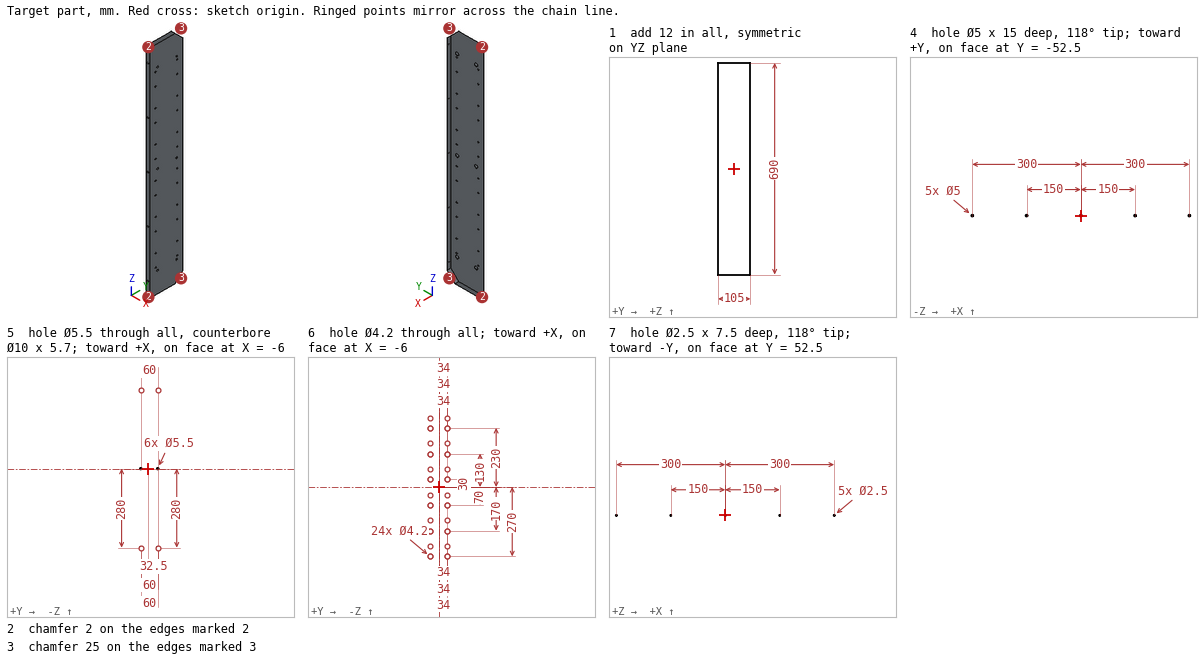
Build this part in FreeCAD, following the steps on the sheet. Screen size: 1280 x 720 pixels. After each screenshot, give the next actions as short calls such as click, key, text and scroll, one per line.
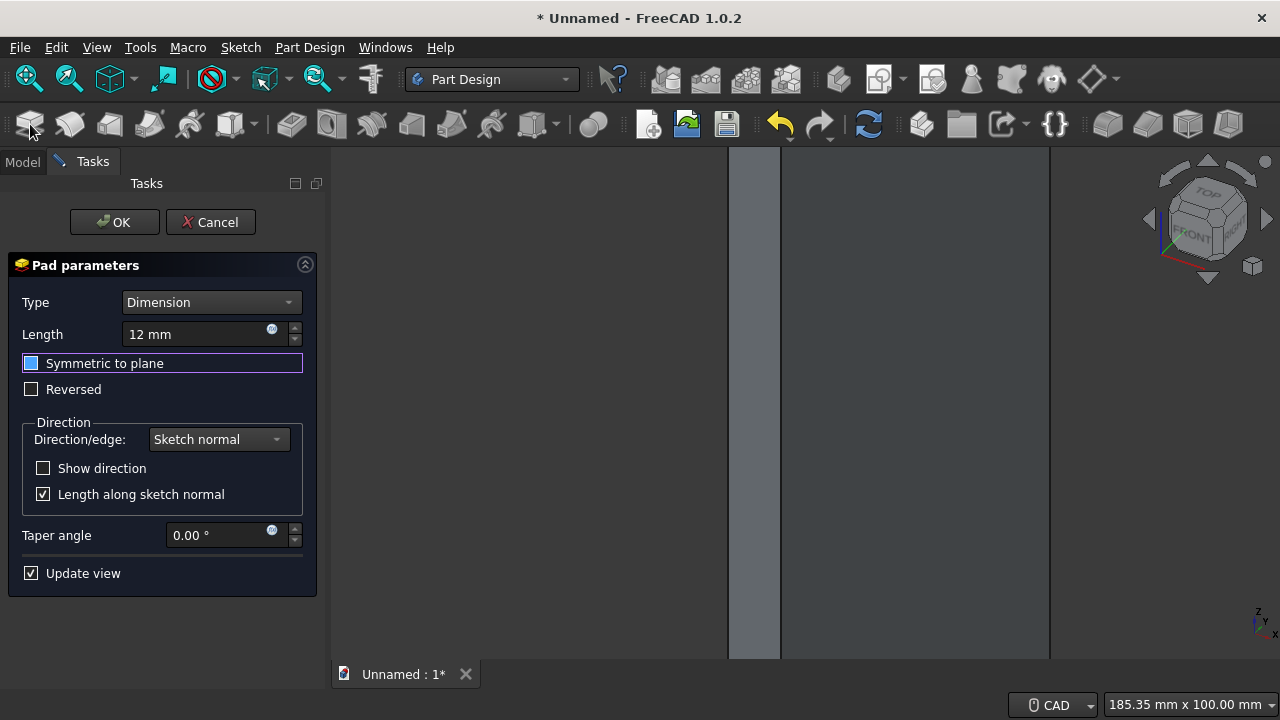
click(30, 363)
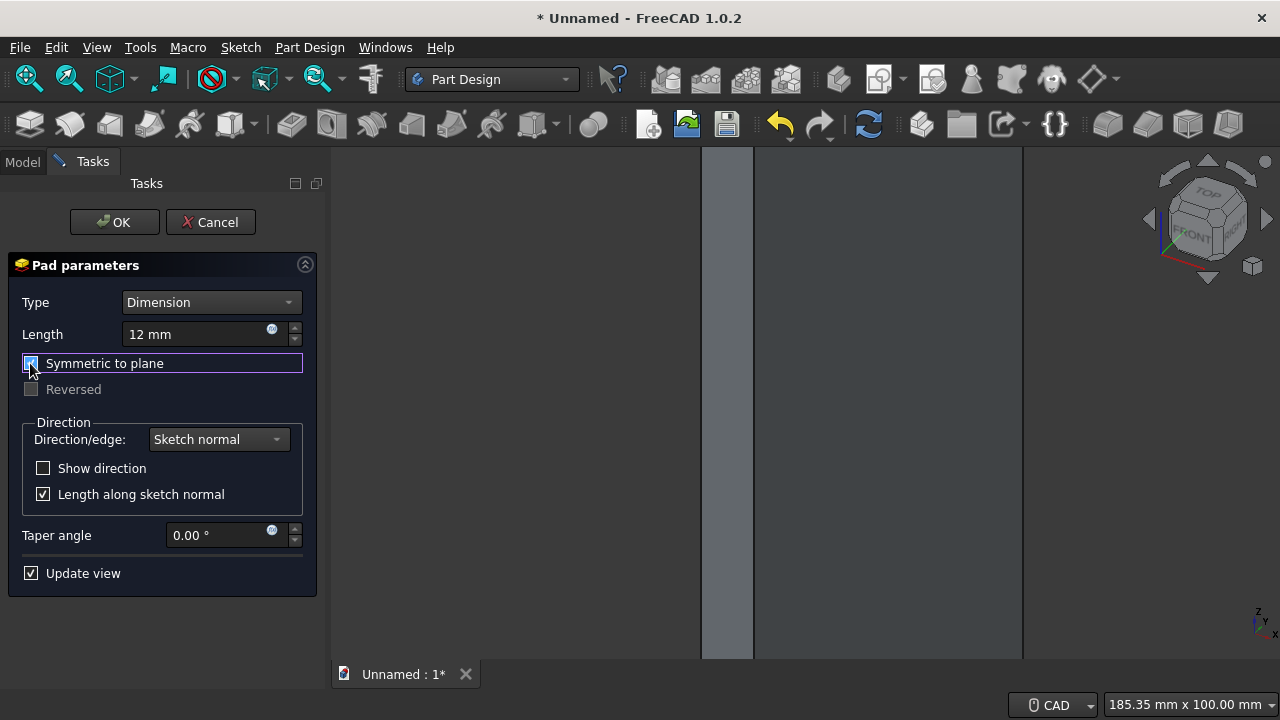
click(115, 222)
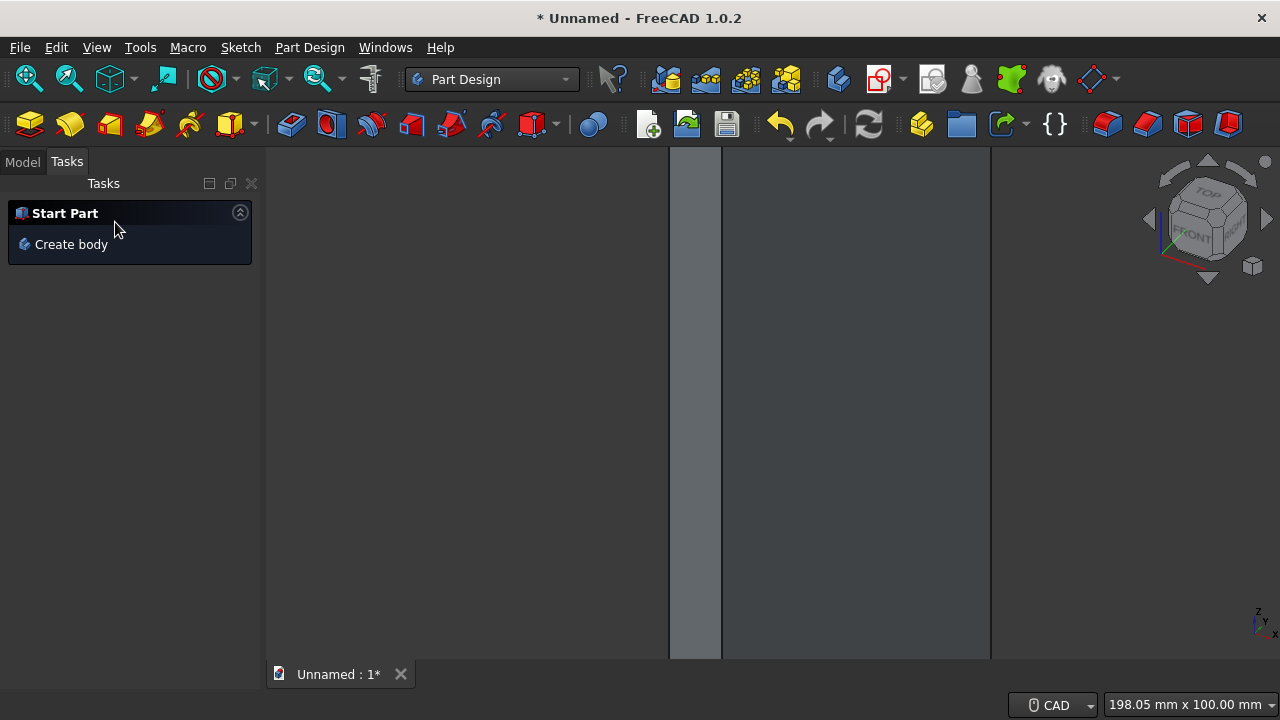
key(v)
key(f)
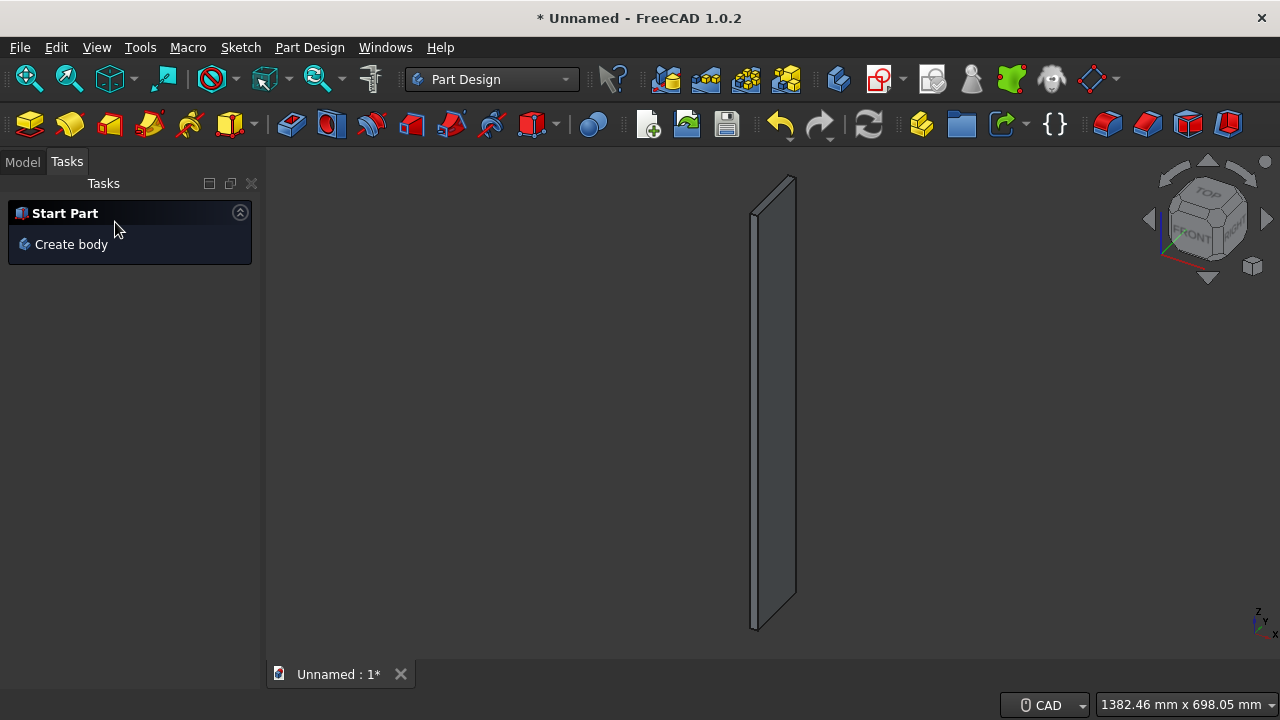
scroll(754, 628, up, 8)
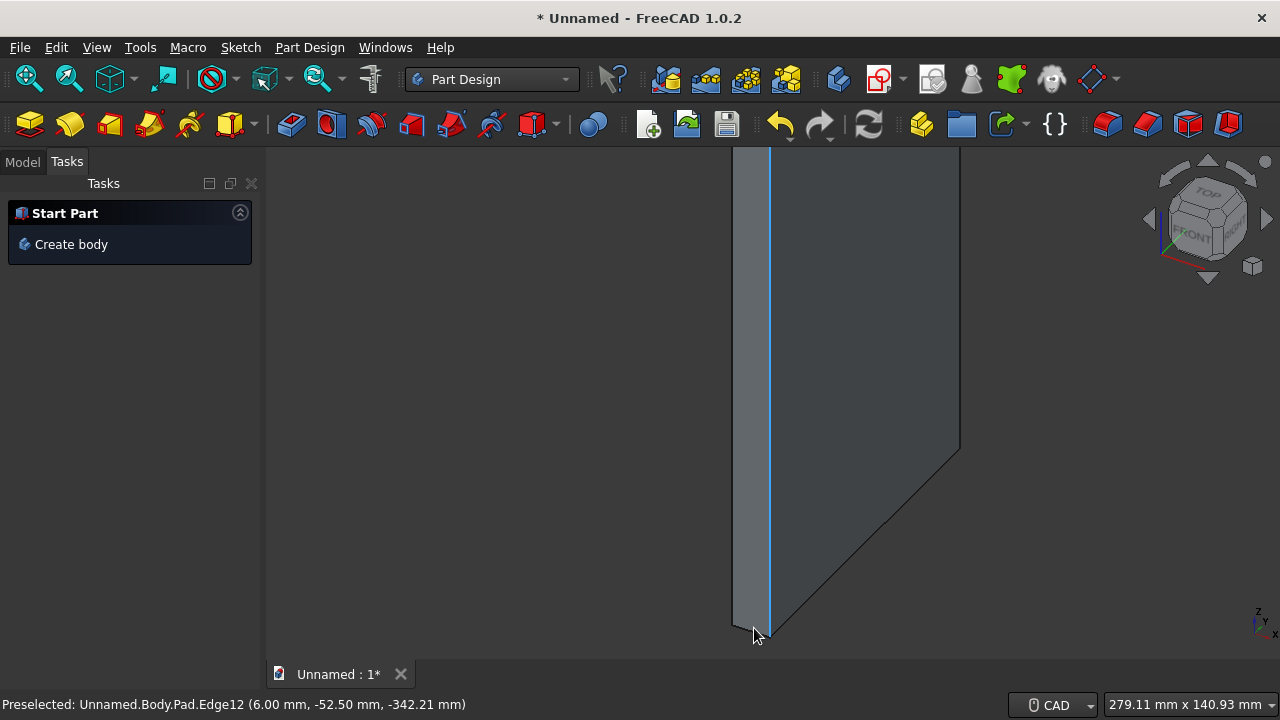
click(30, 80)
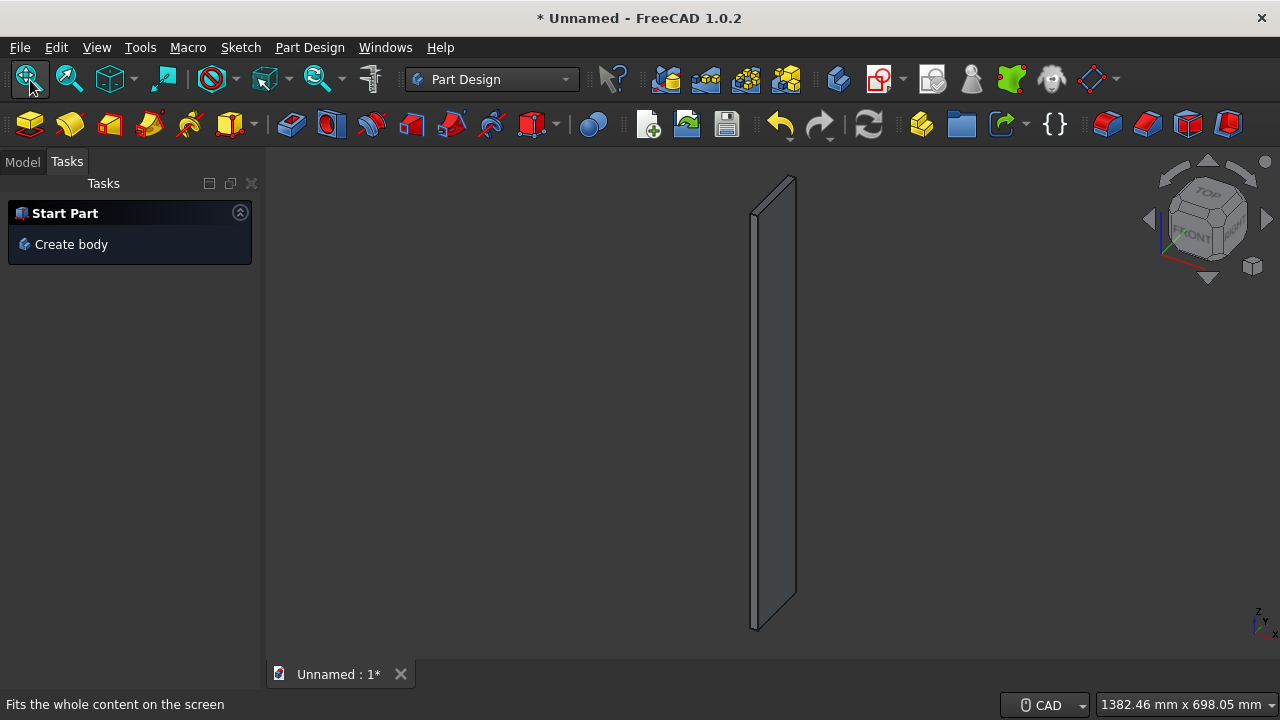
key(0)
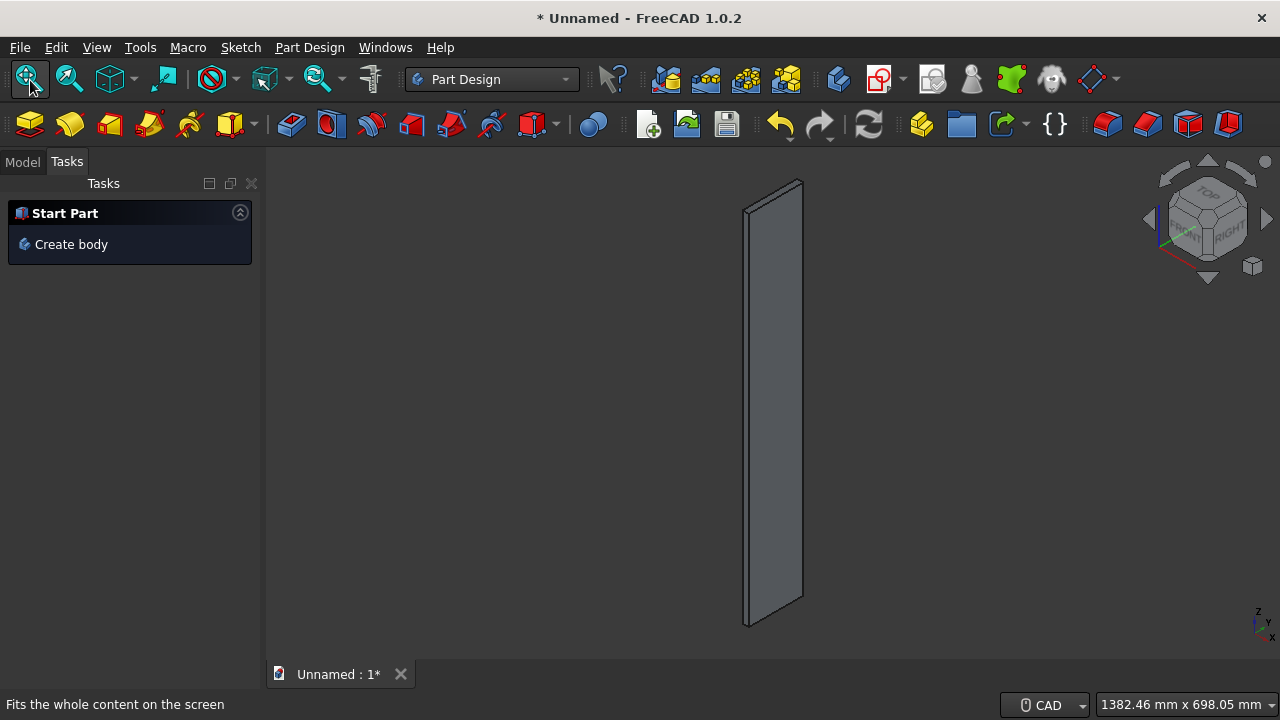
scroll(746, 624, up, 8)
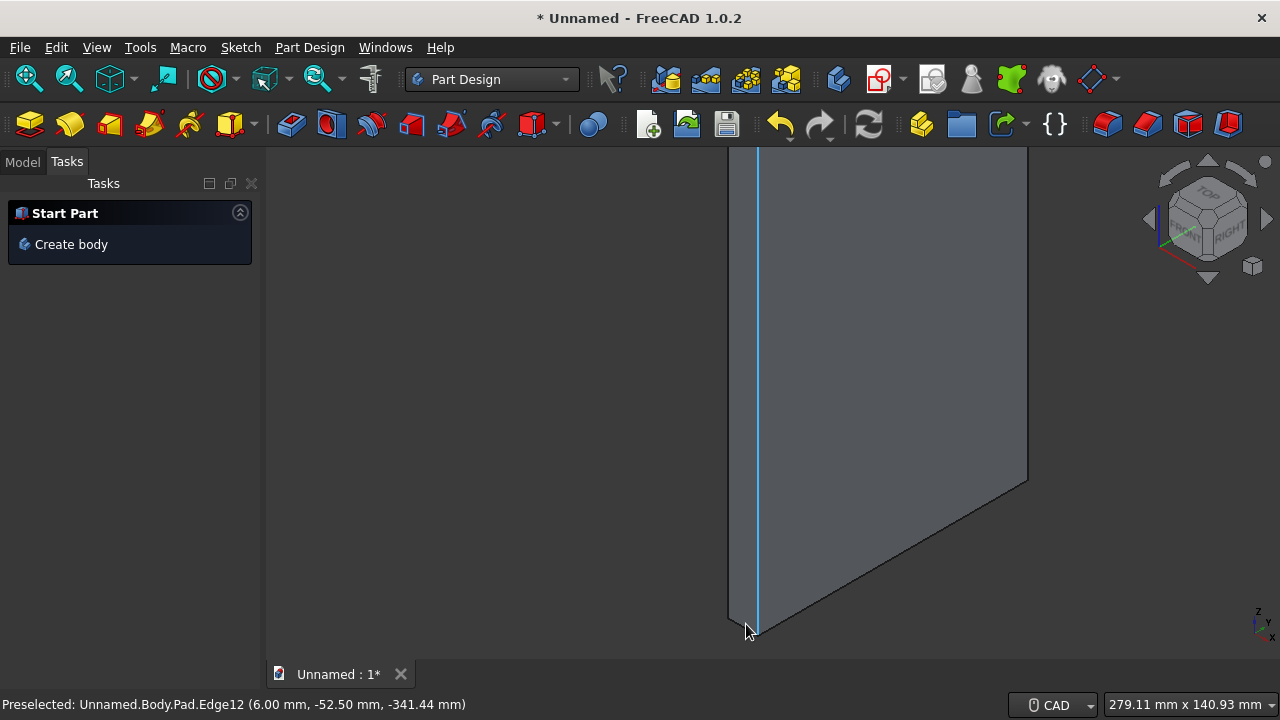
click(30, 80)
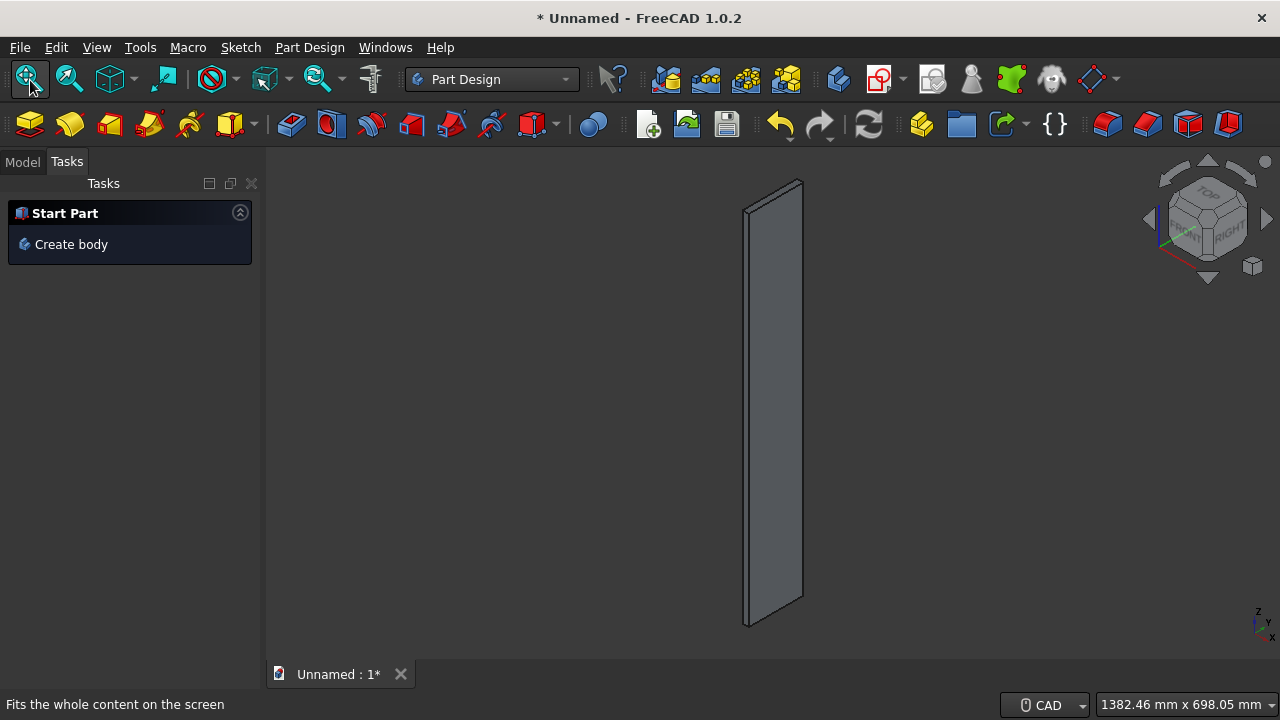
key(2)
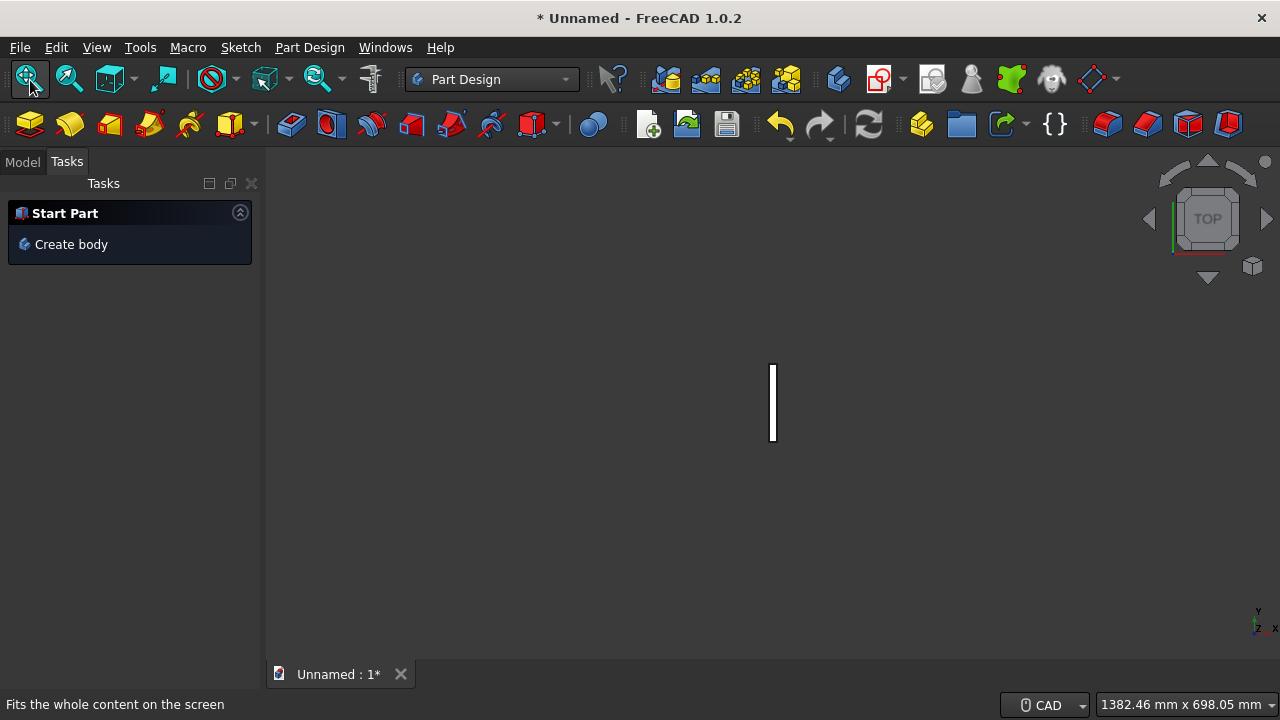
click(30, 80)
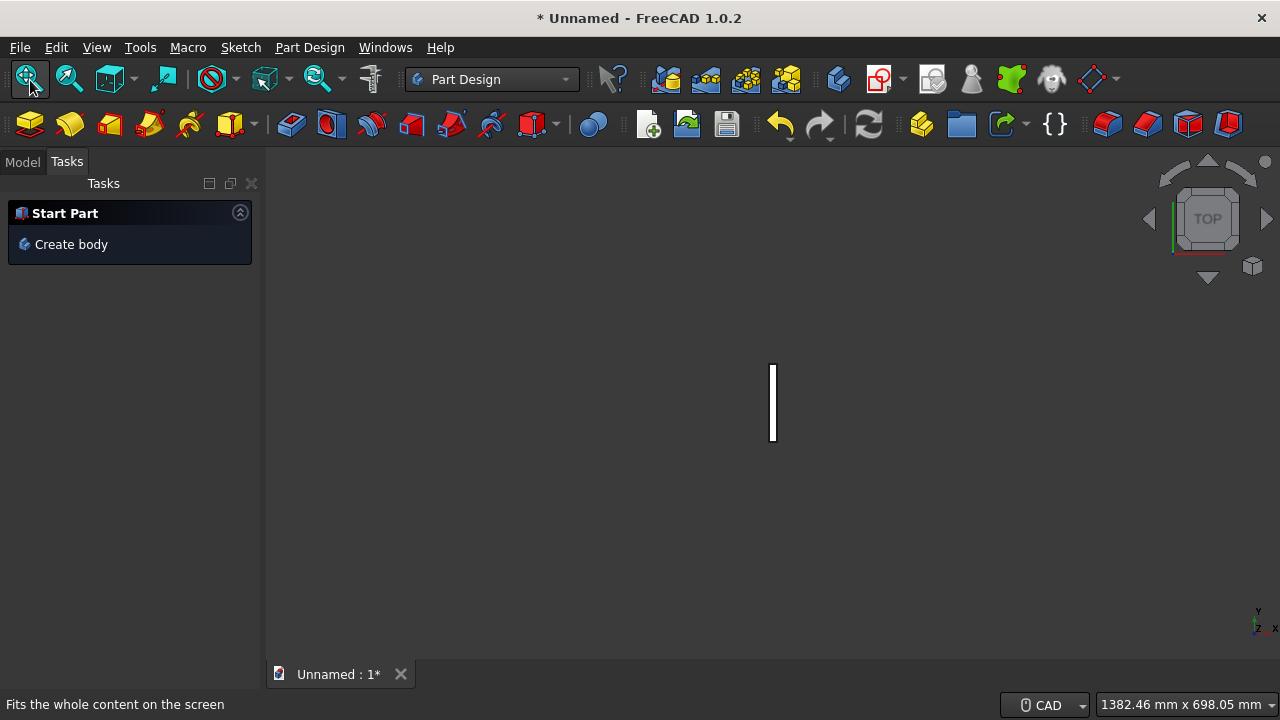
scroll(773, 441, up, 8)